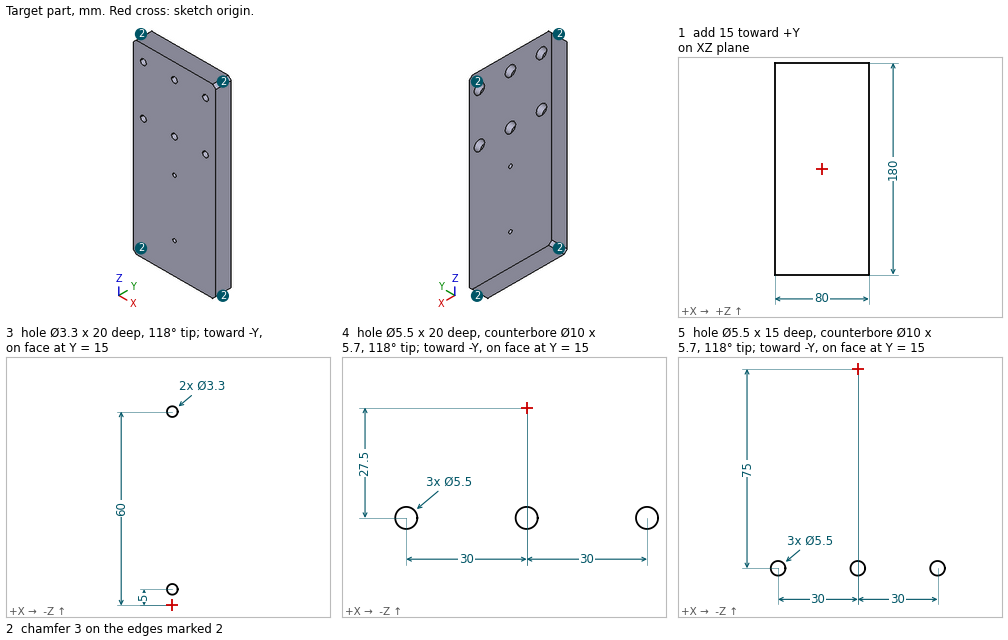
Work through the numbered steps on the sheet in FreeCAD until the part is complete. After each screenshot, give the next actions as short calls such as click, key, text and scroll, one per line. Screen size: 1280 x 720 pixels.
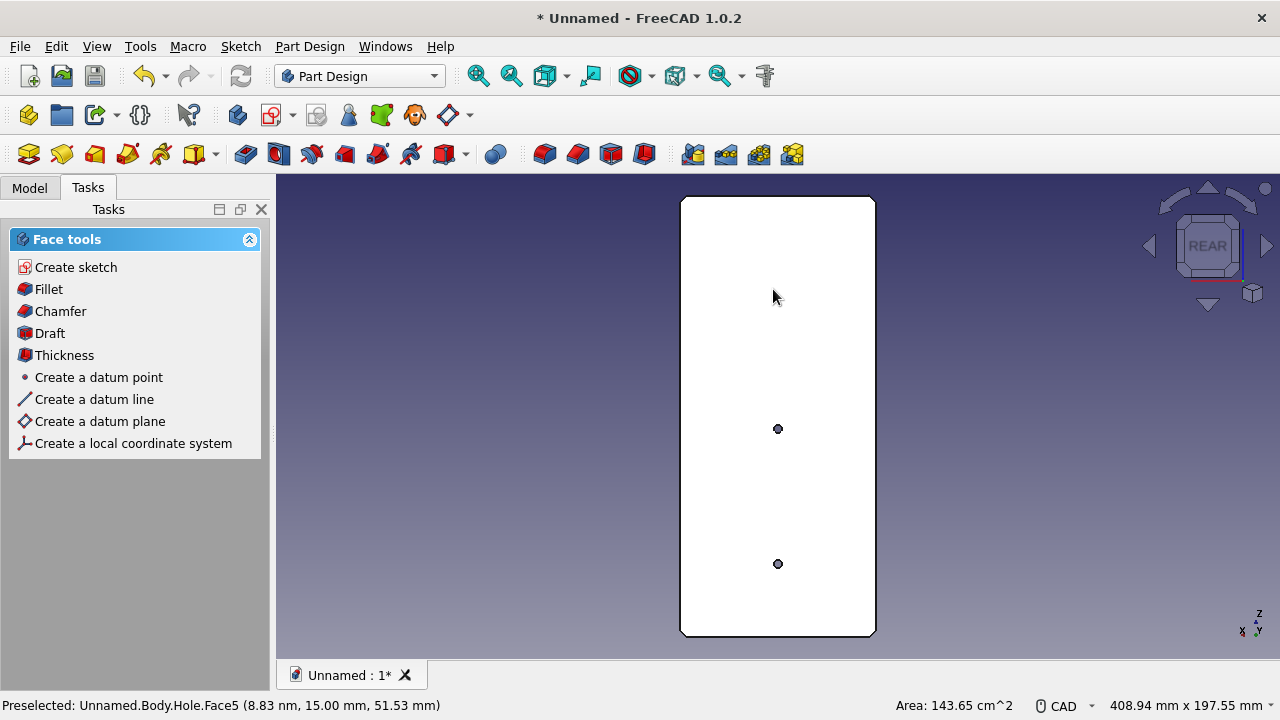
click(270, 116)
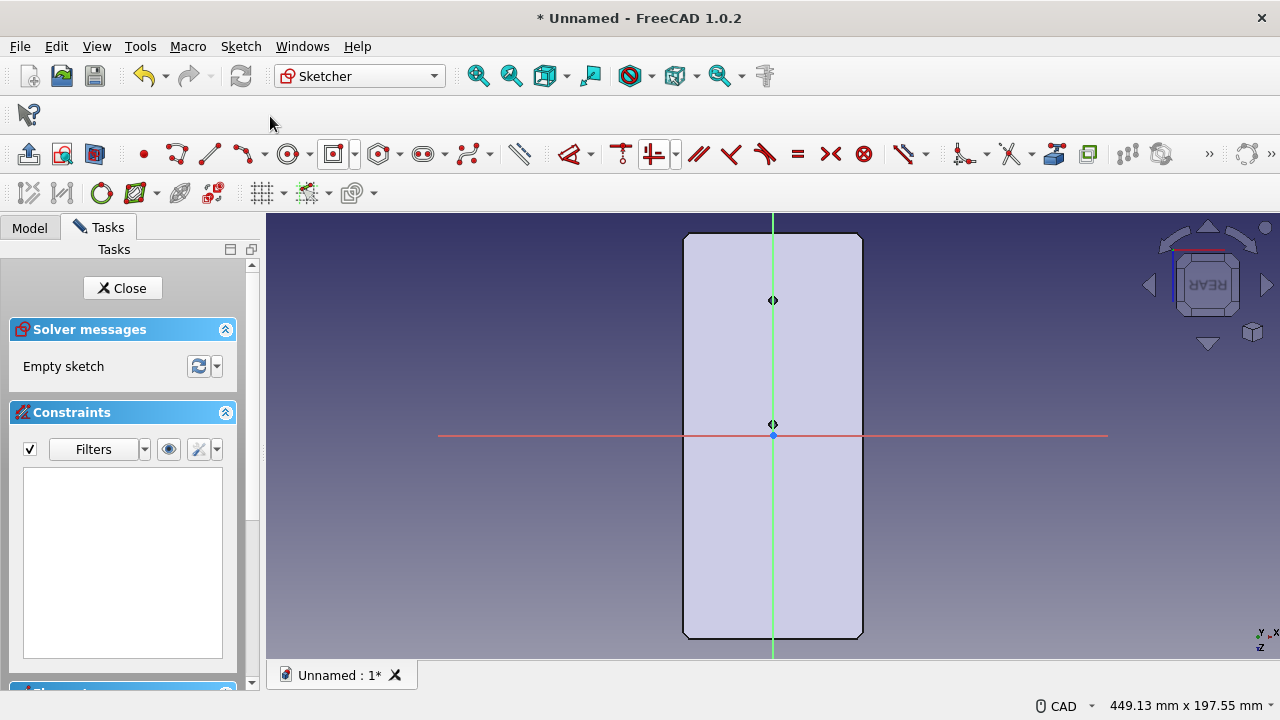
scroll(795, 481, up, 7)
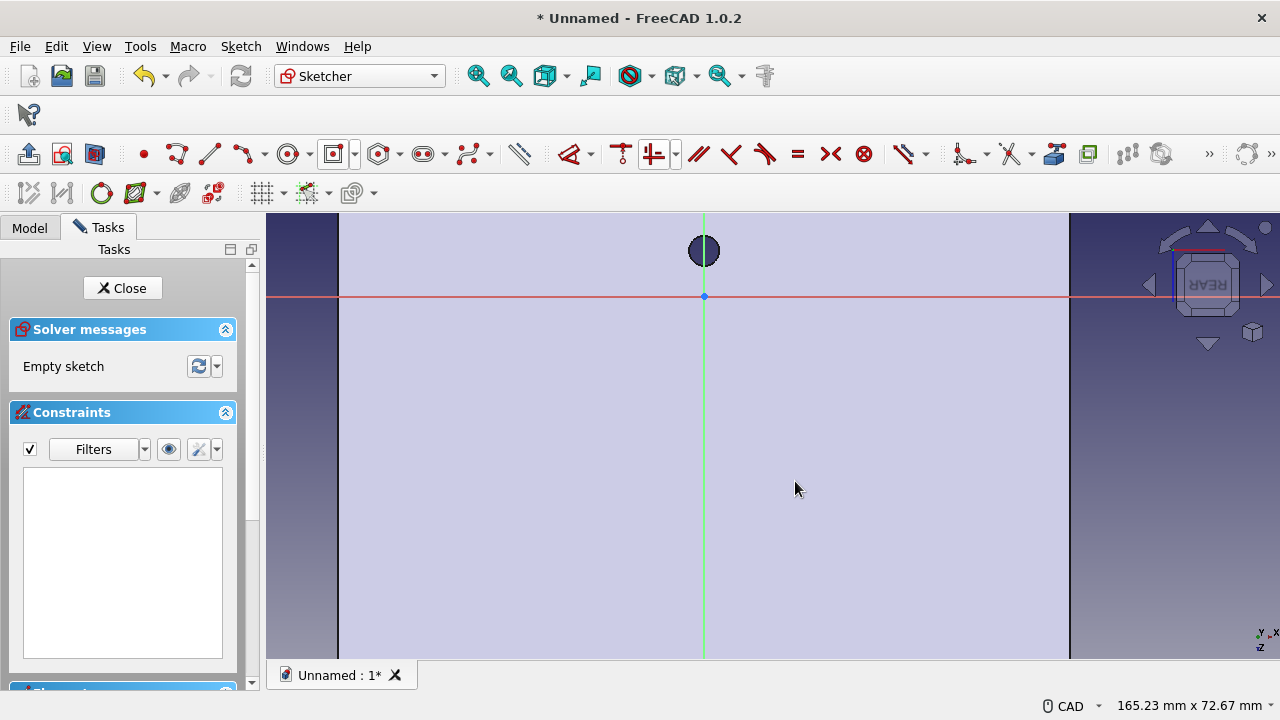
click(288, 154)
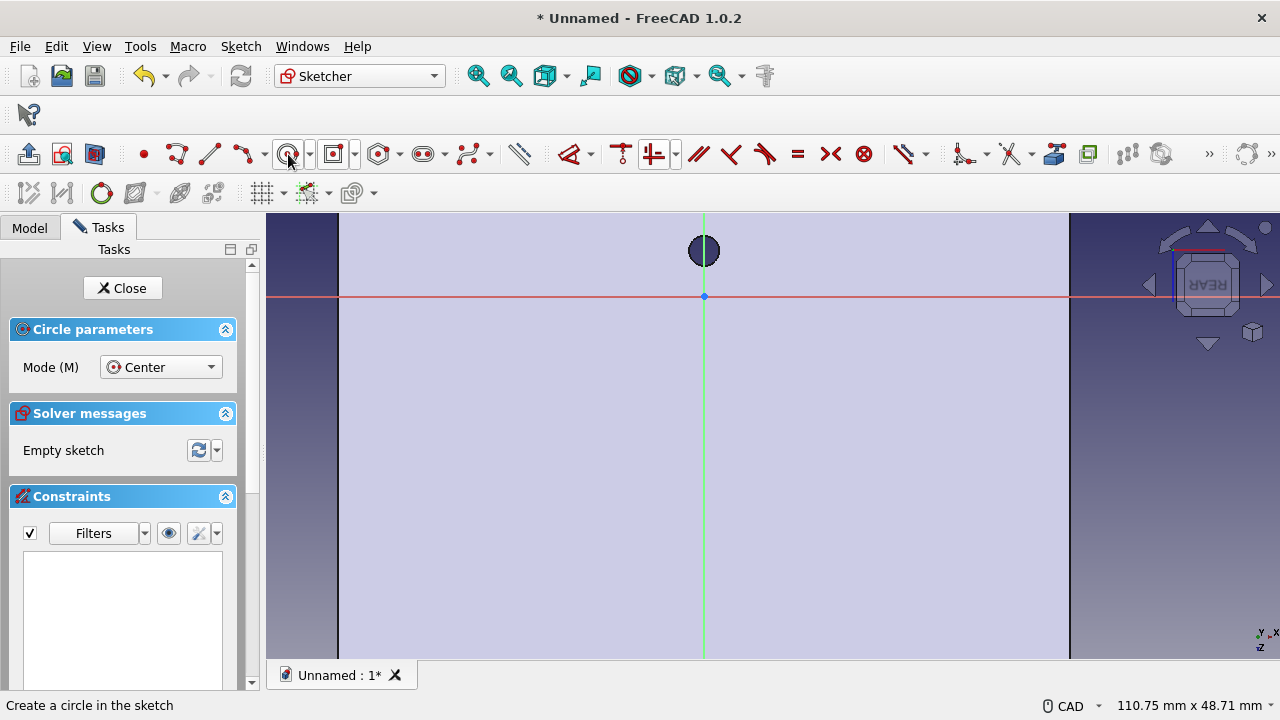
click(430, 548)
click(447, 531)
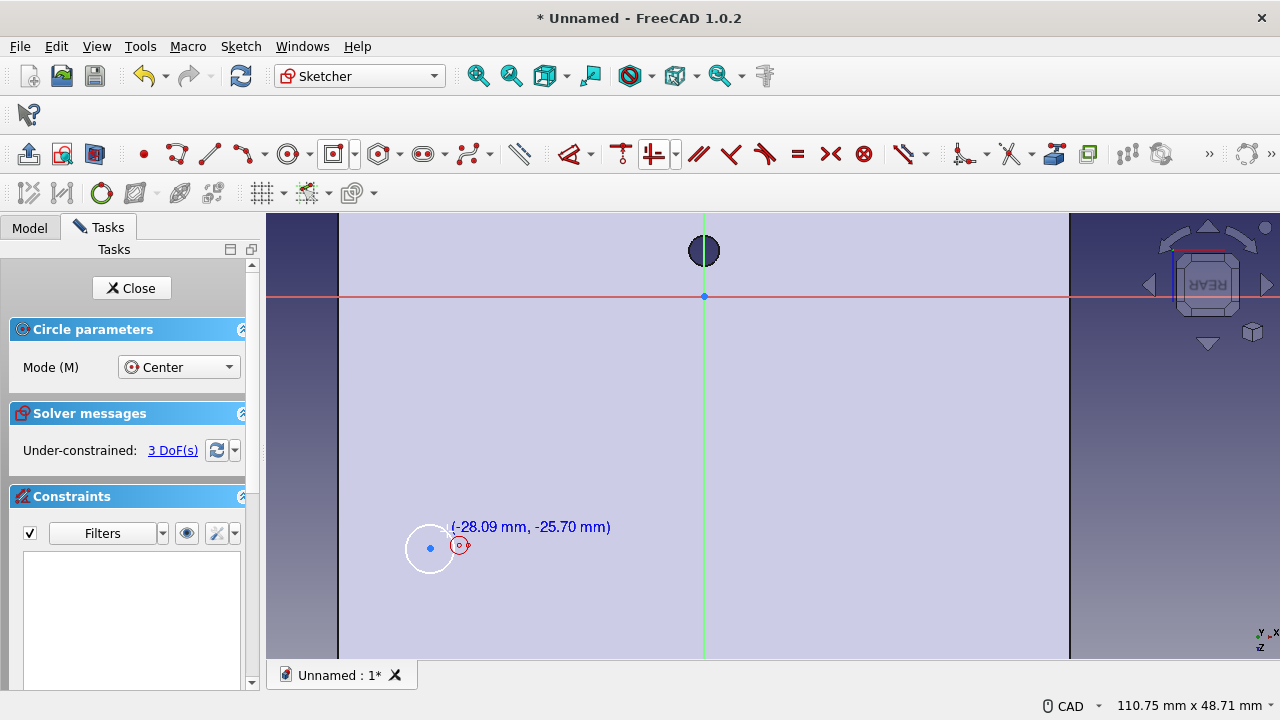
click(704, 548)
click(722, 531)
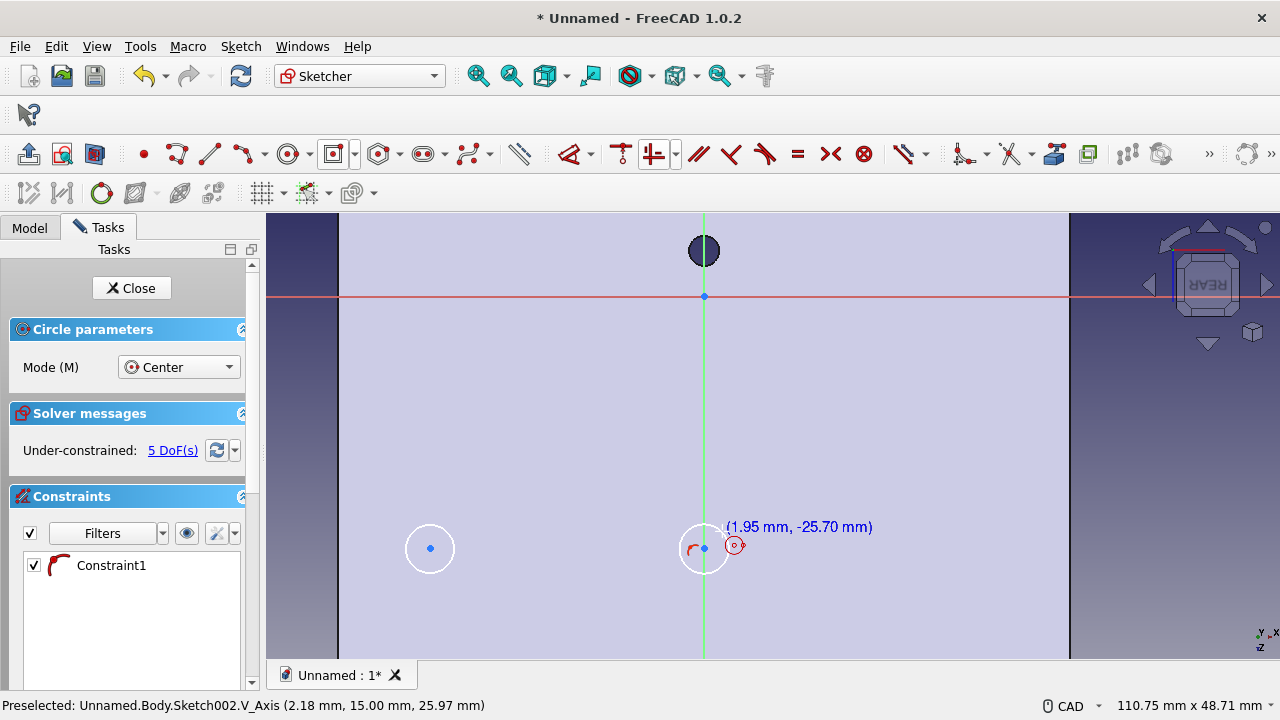
click(979, 548)
click(997, 531)
key(Escape)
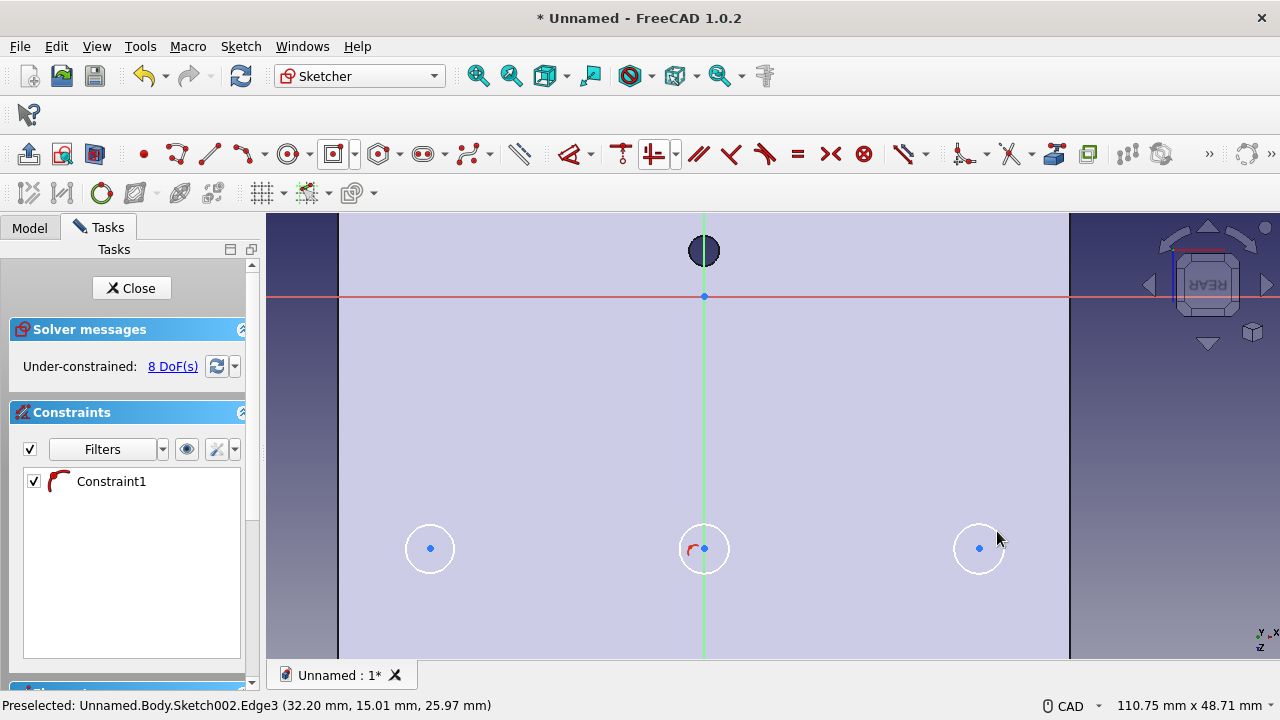
click(447, 532)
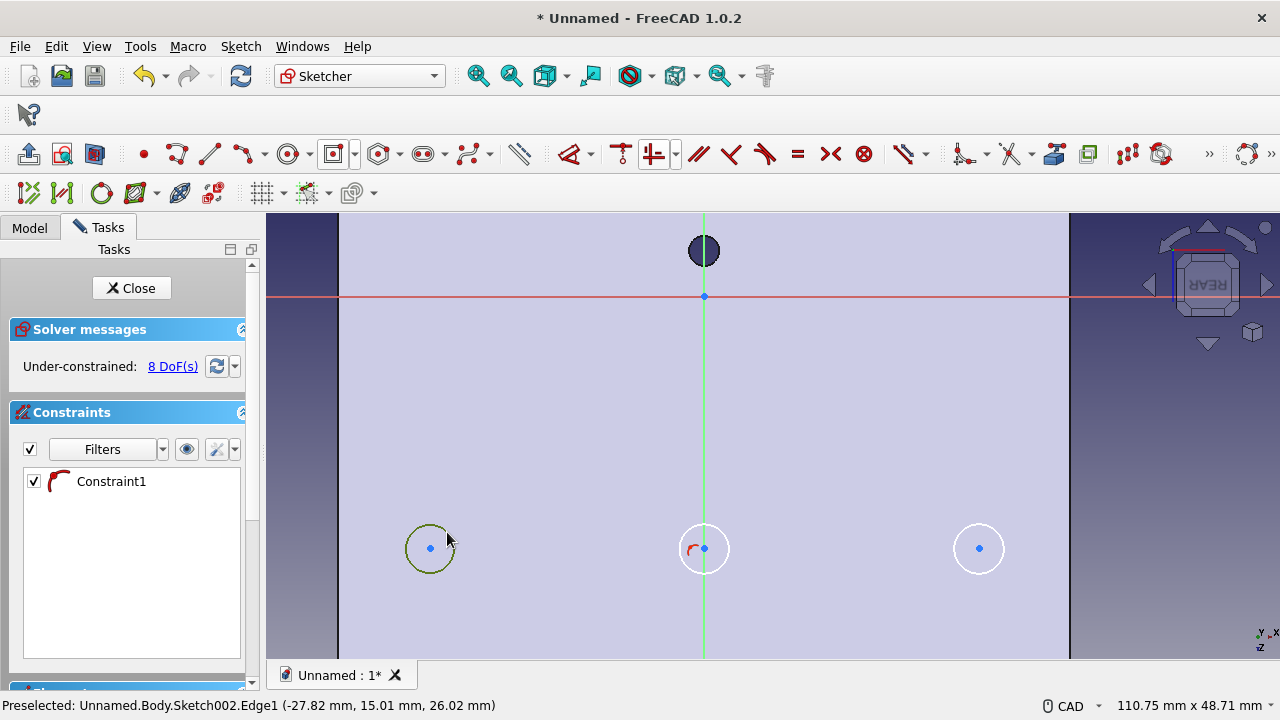
click(722, 532)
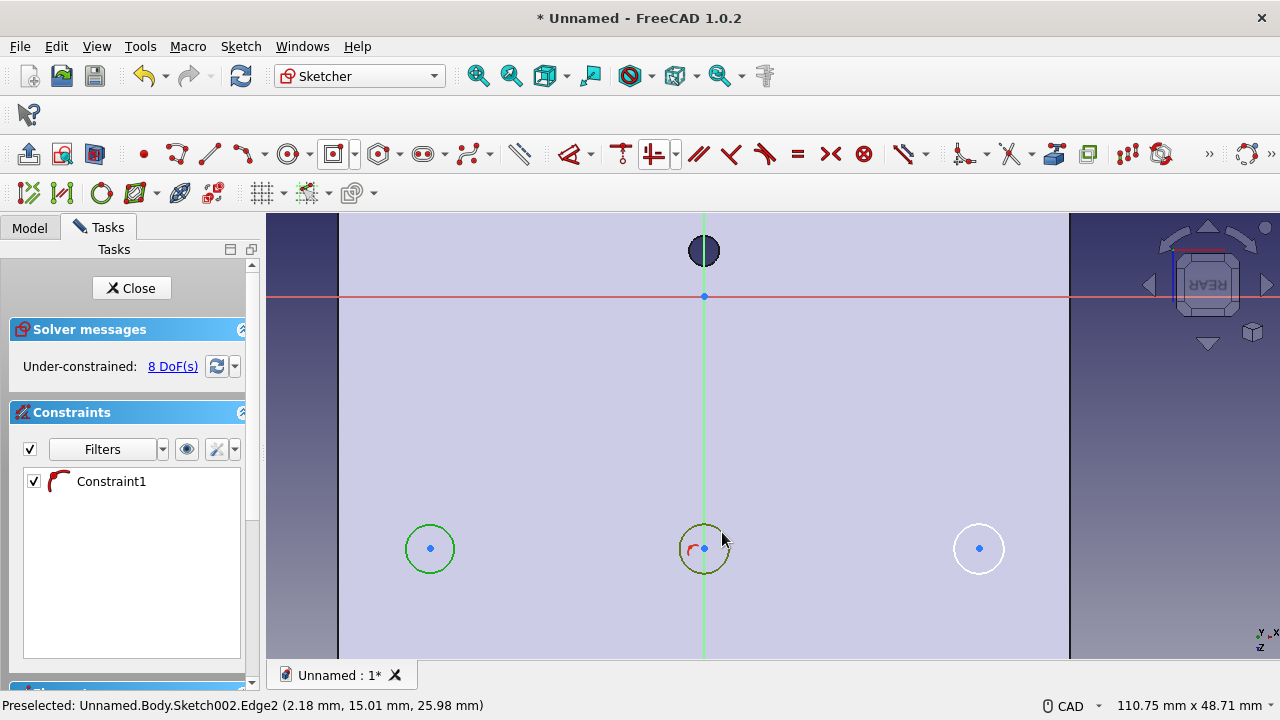
click(996, 531)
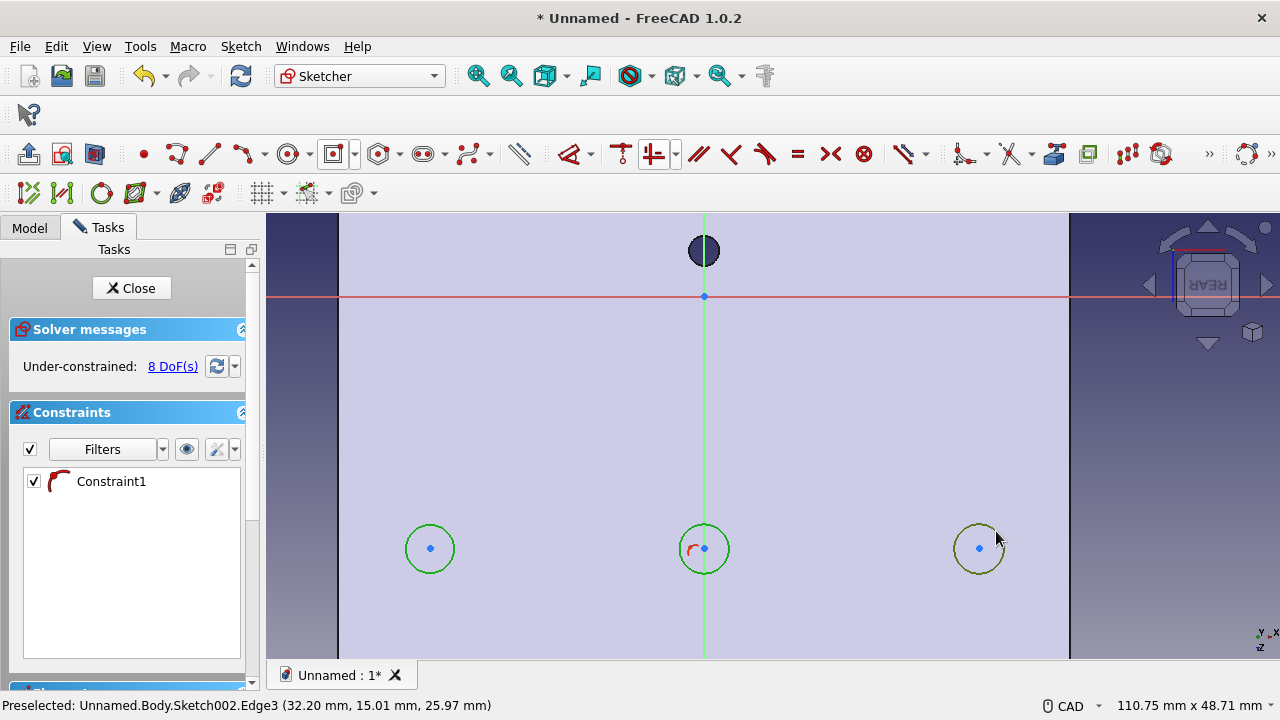
click(798, 154)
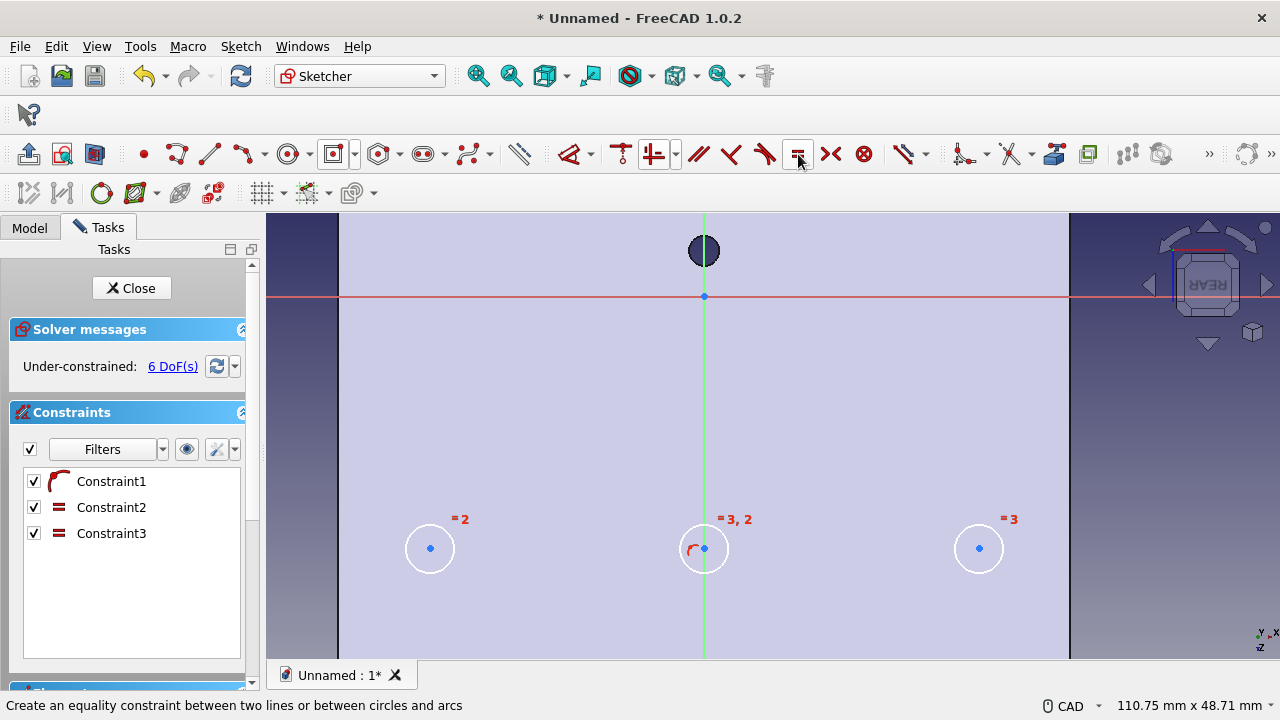
click(430, 549)